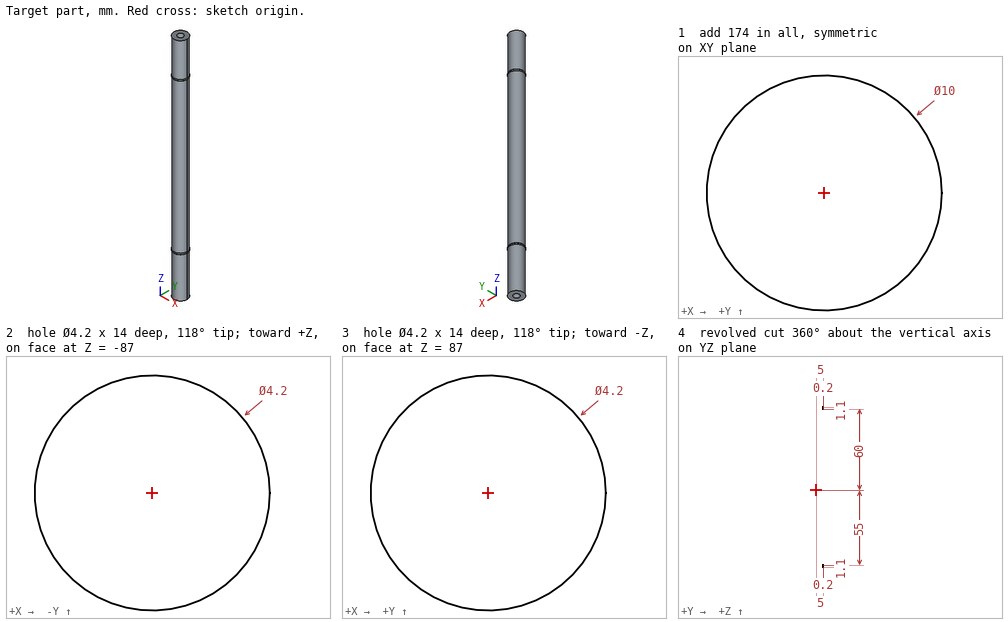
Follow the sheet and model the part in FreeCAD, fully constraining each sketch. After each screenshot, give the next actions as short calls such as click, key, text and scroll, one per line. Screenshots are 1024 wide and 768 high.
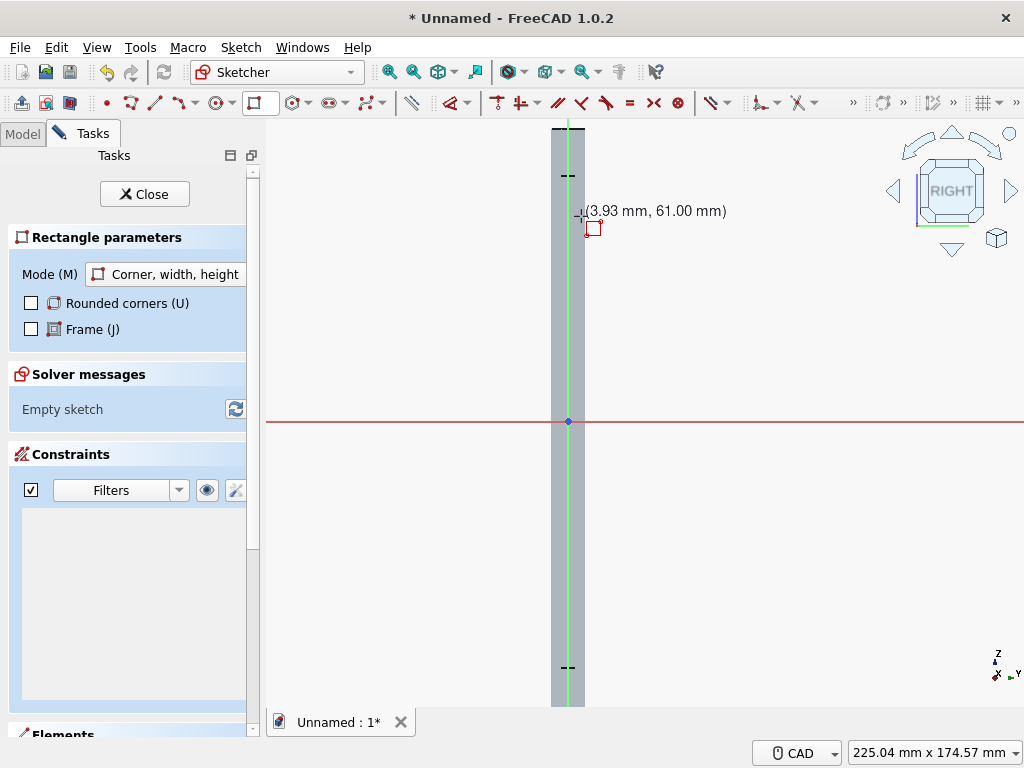
click(584, 216)
click(585, 220)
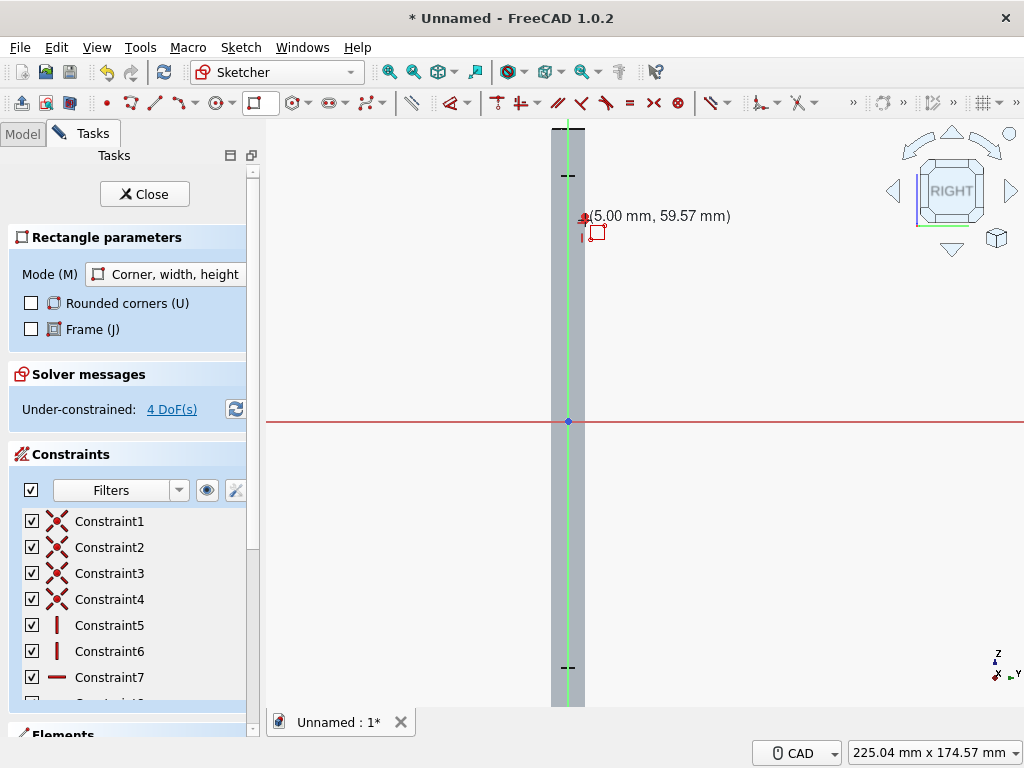
scroll(584, 607, up, 16)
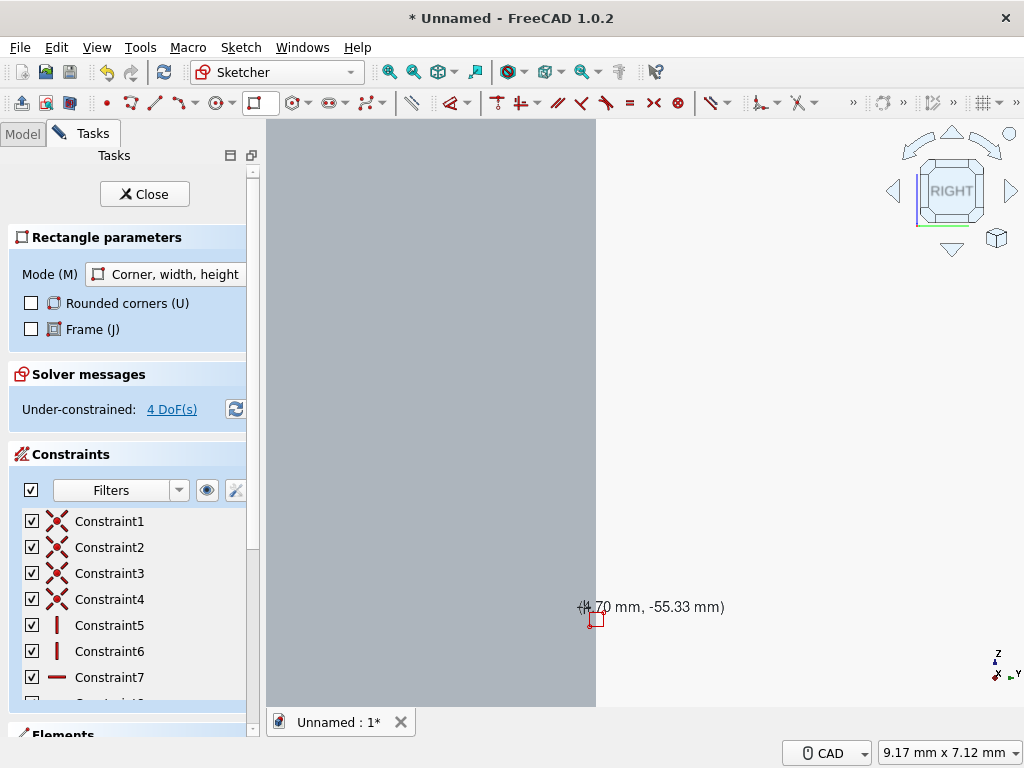
scroll(584, 608, down, 16)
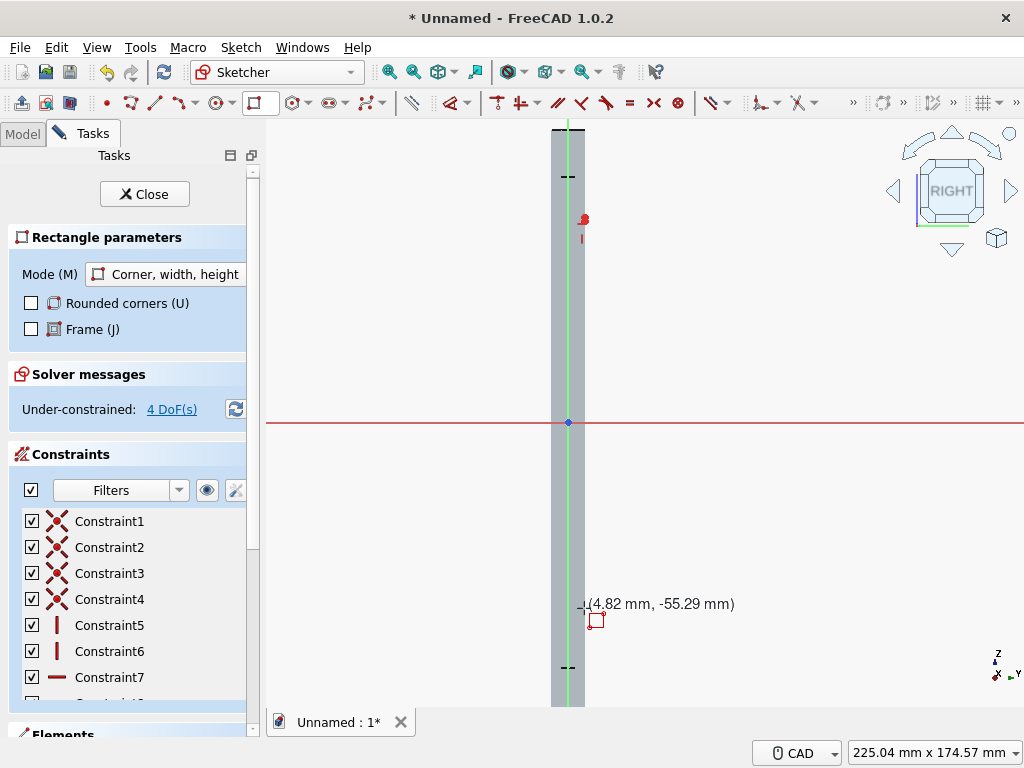
click(584, 608)
click(585, 612)
key(Escape)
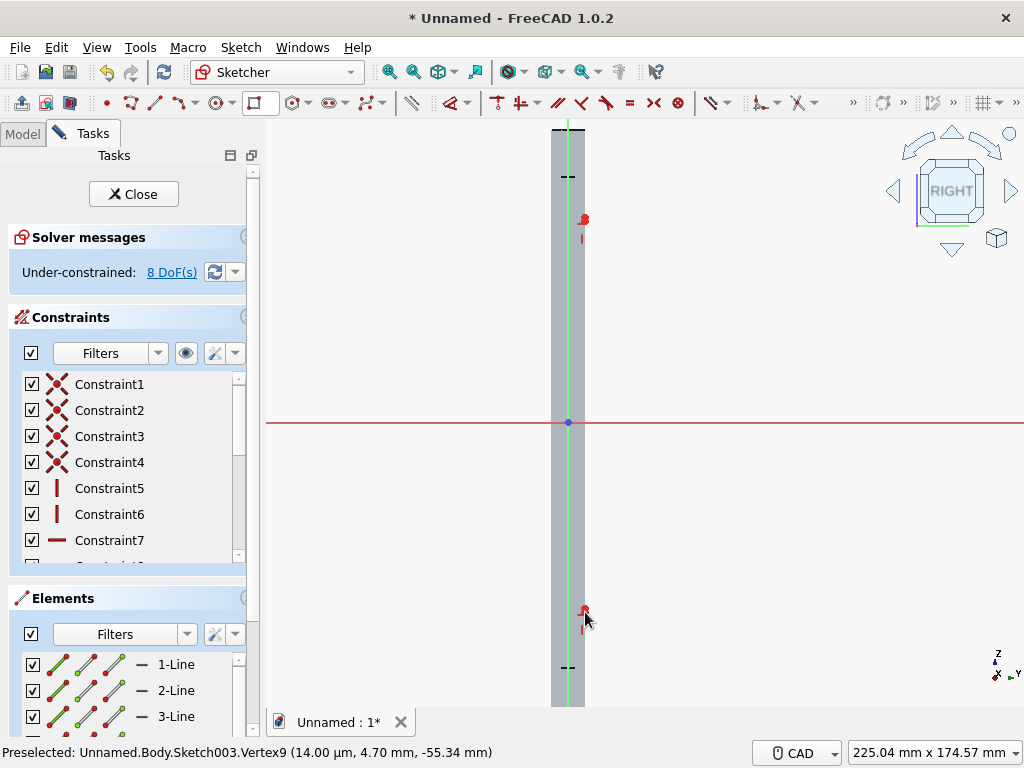
click(450, 104)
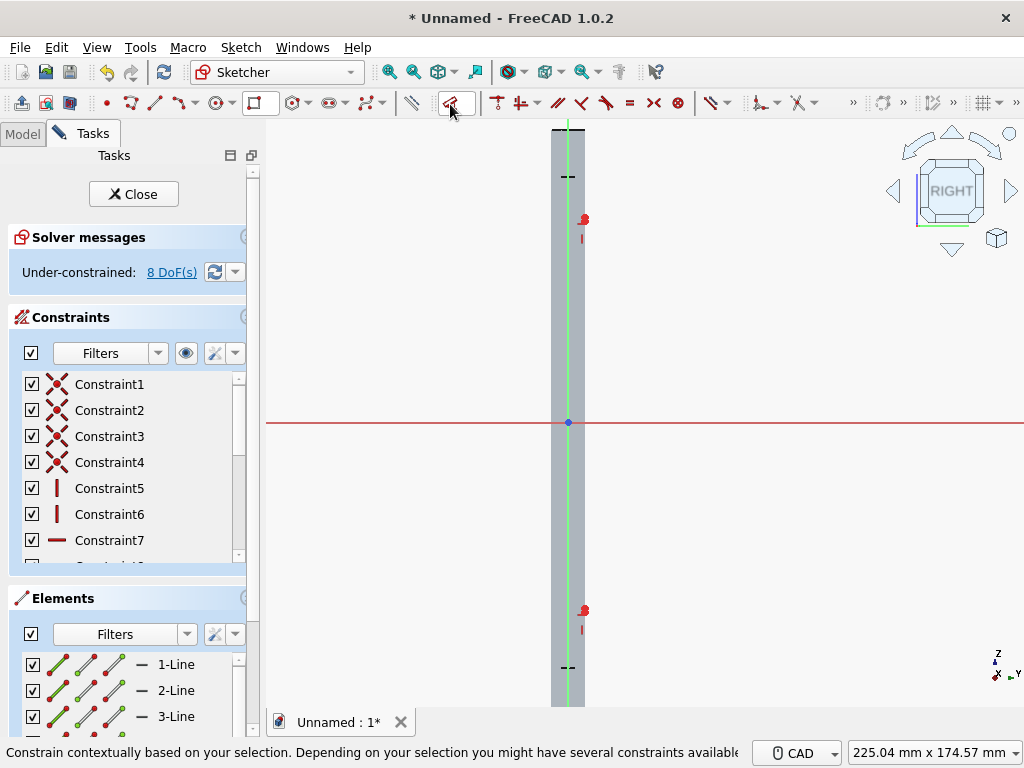
scroll(585, 222, up, 13)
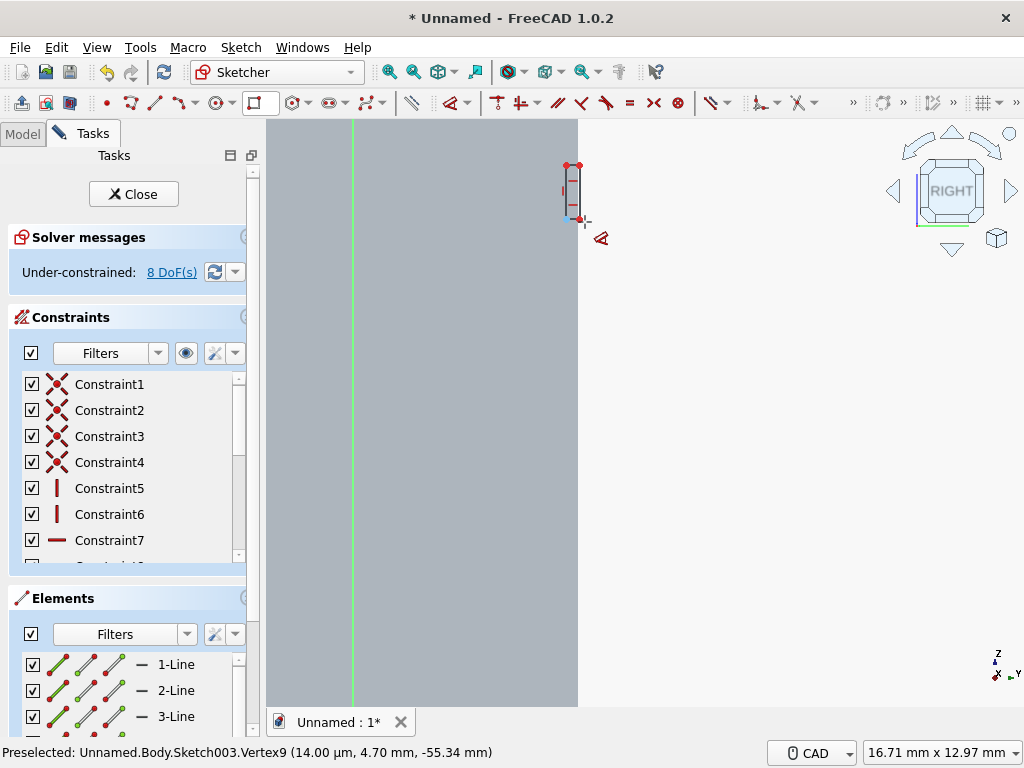
click(580, 219)
click(466, 185)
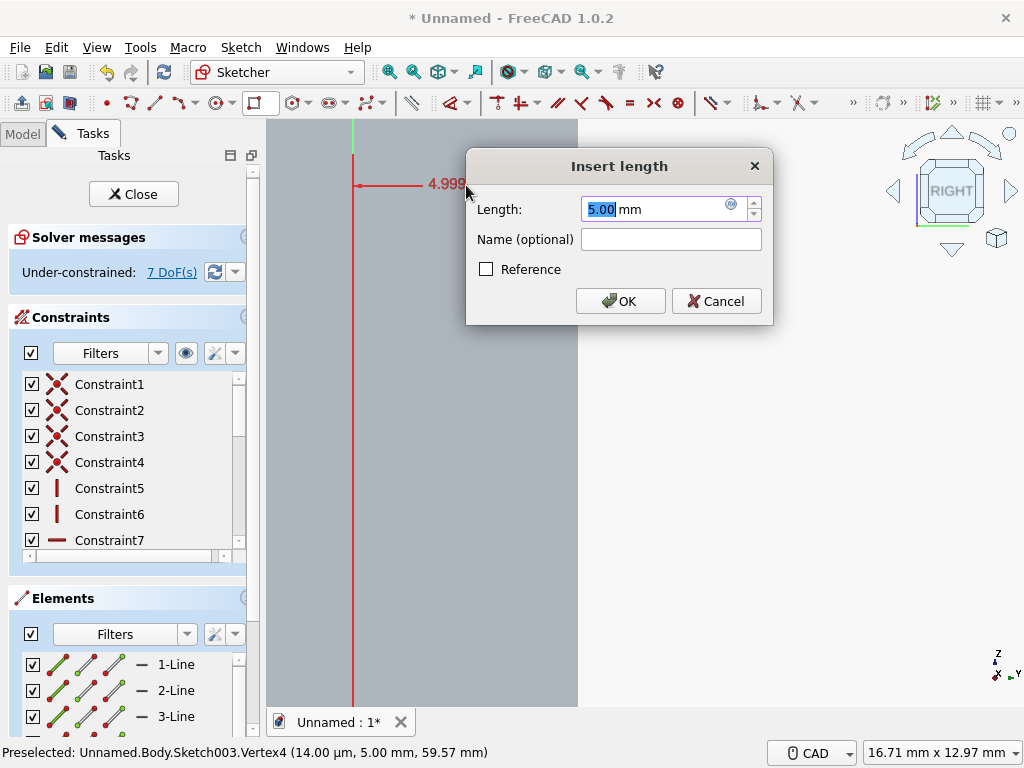
text(5)
key(Return)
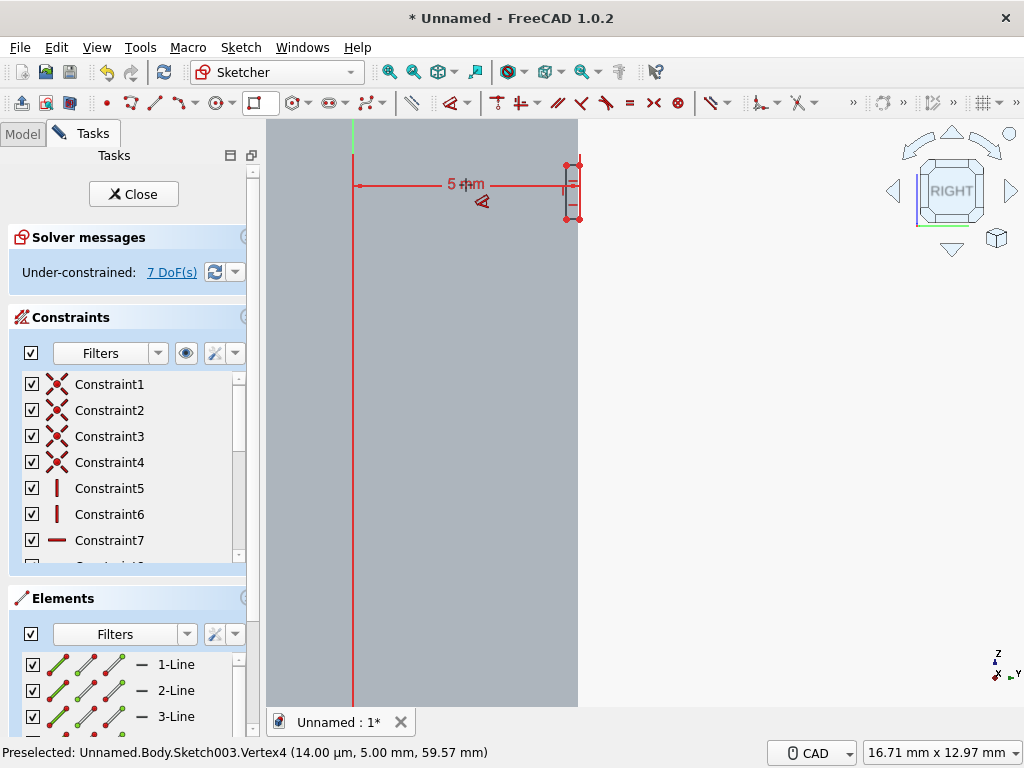
scroll(585, 221, down, 13)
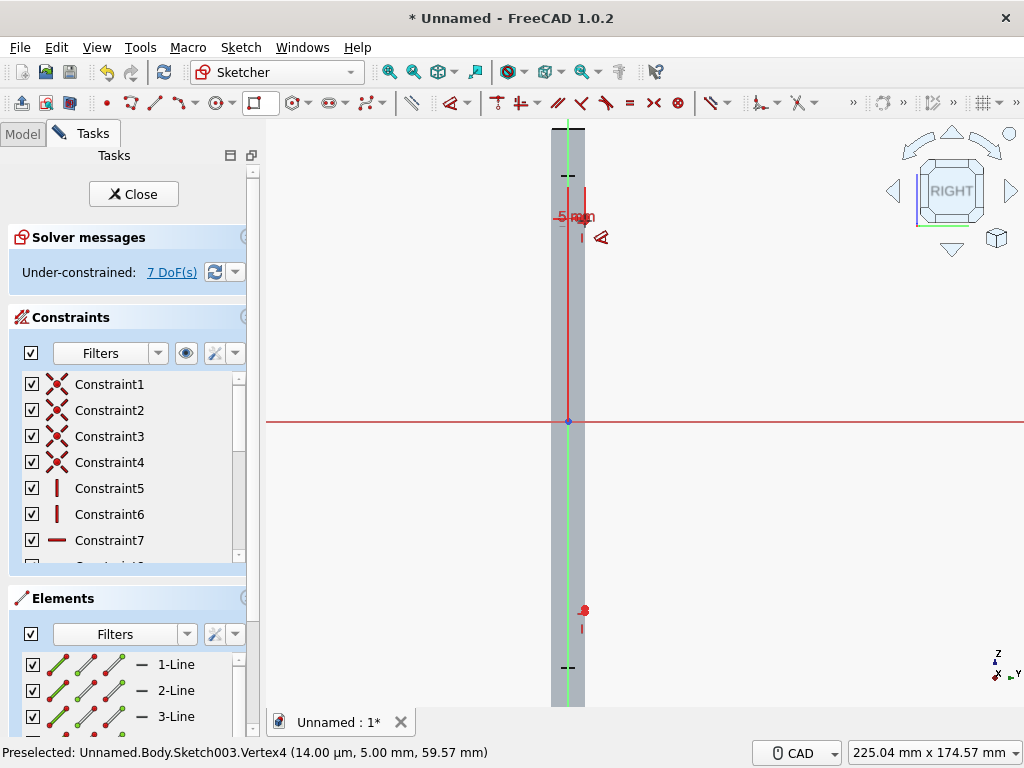
scroll(585, 612, up, 13)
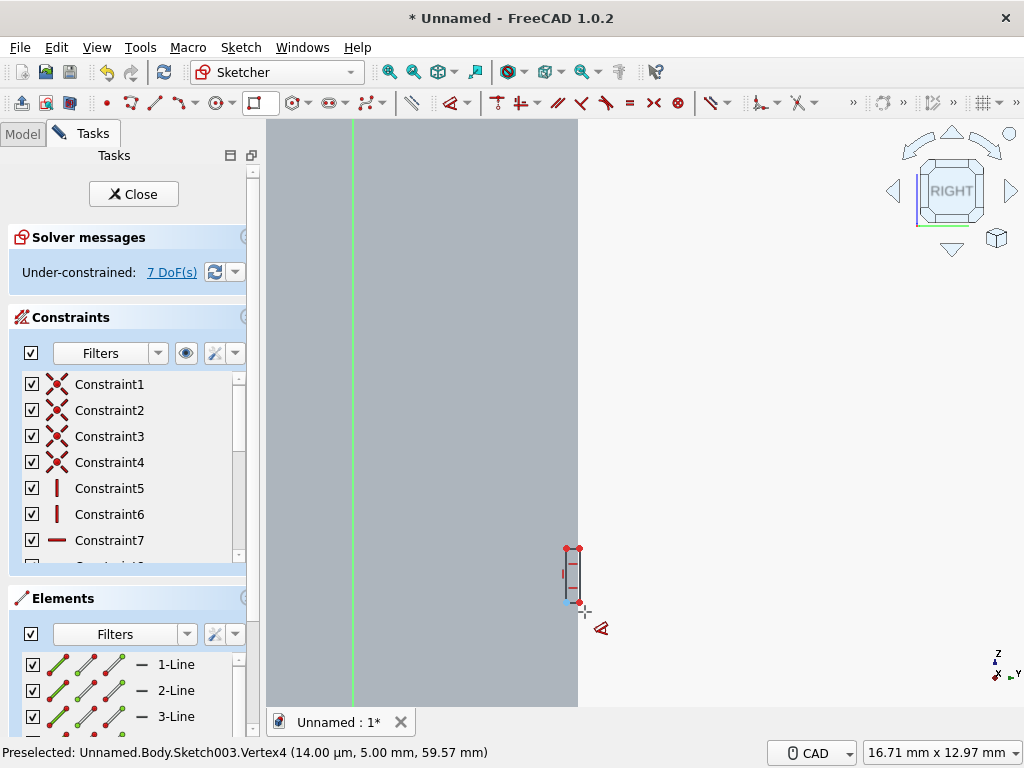
click(580, 603)
click(466, 637)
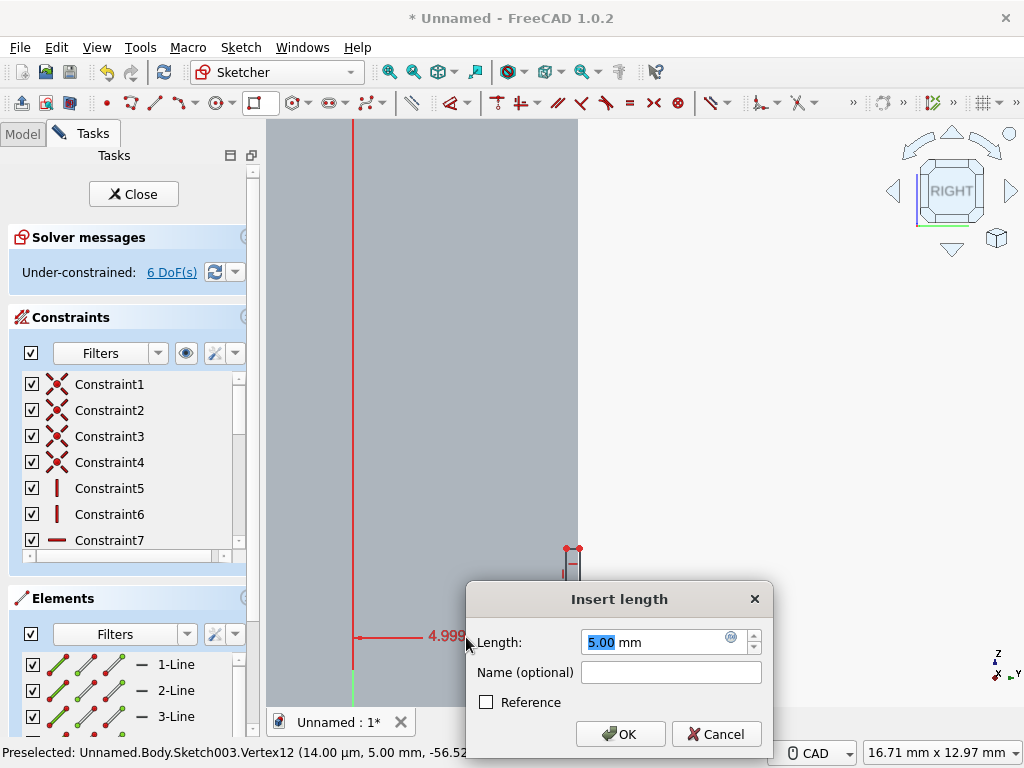
text(5)
key(Return)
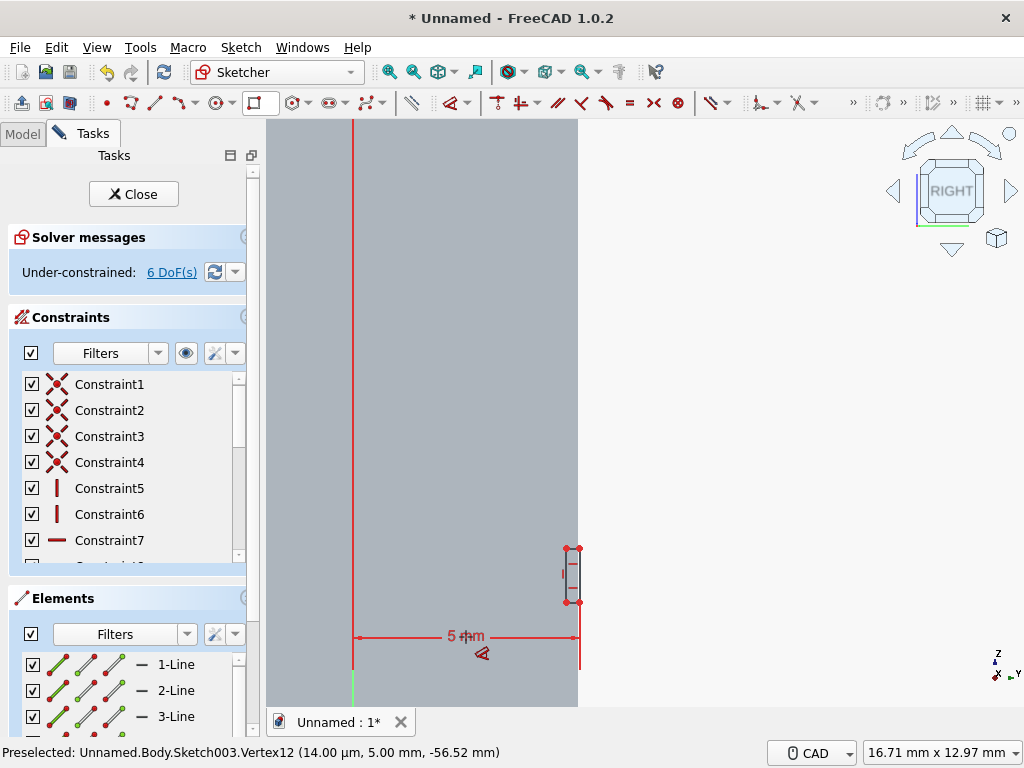
scroll(585, 613, down, 13)